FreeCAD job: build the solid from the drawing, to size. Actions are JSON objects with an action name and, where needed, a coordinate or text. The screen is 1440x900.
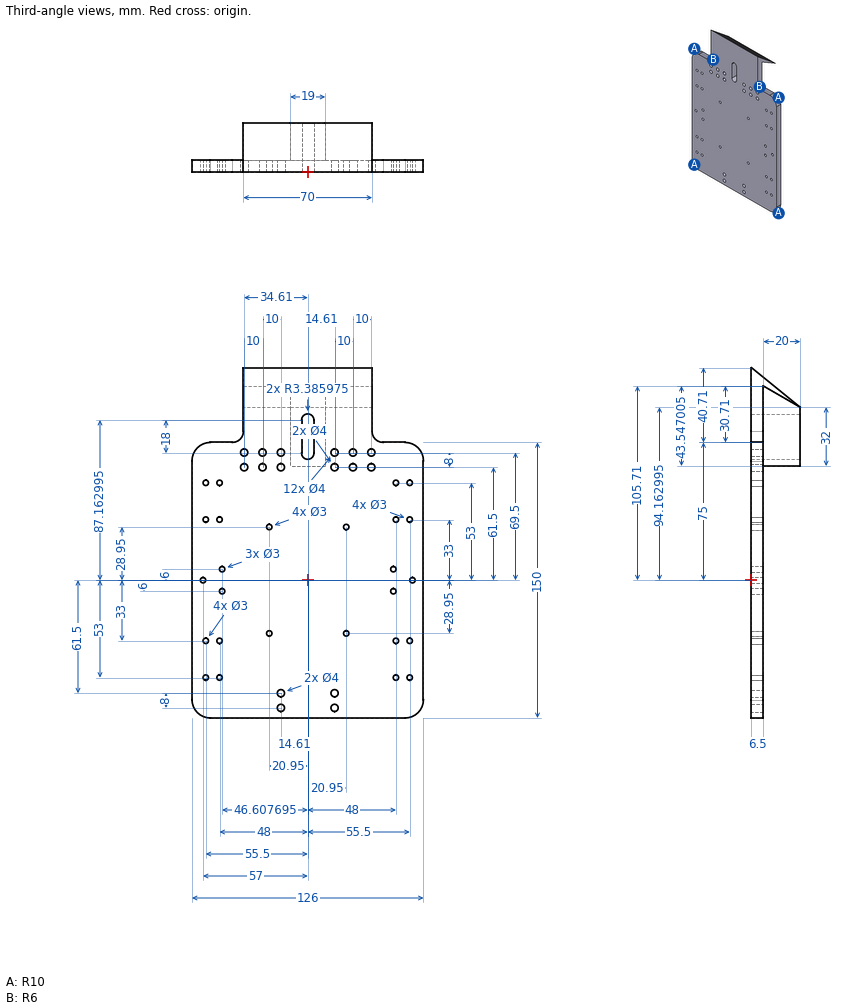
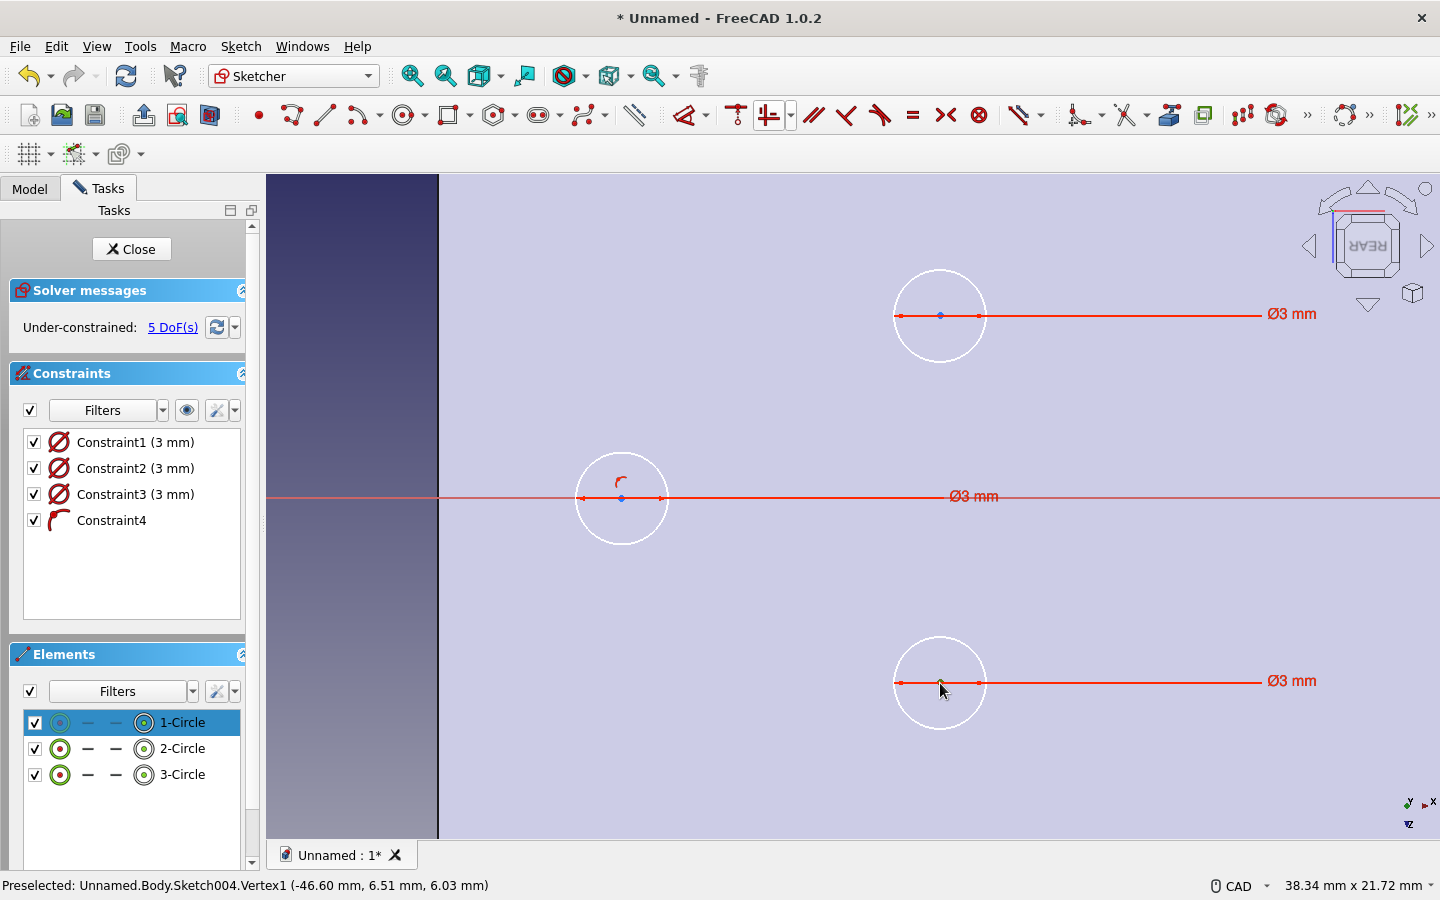
{"action": "left_click", "coordinate": [940, 316]}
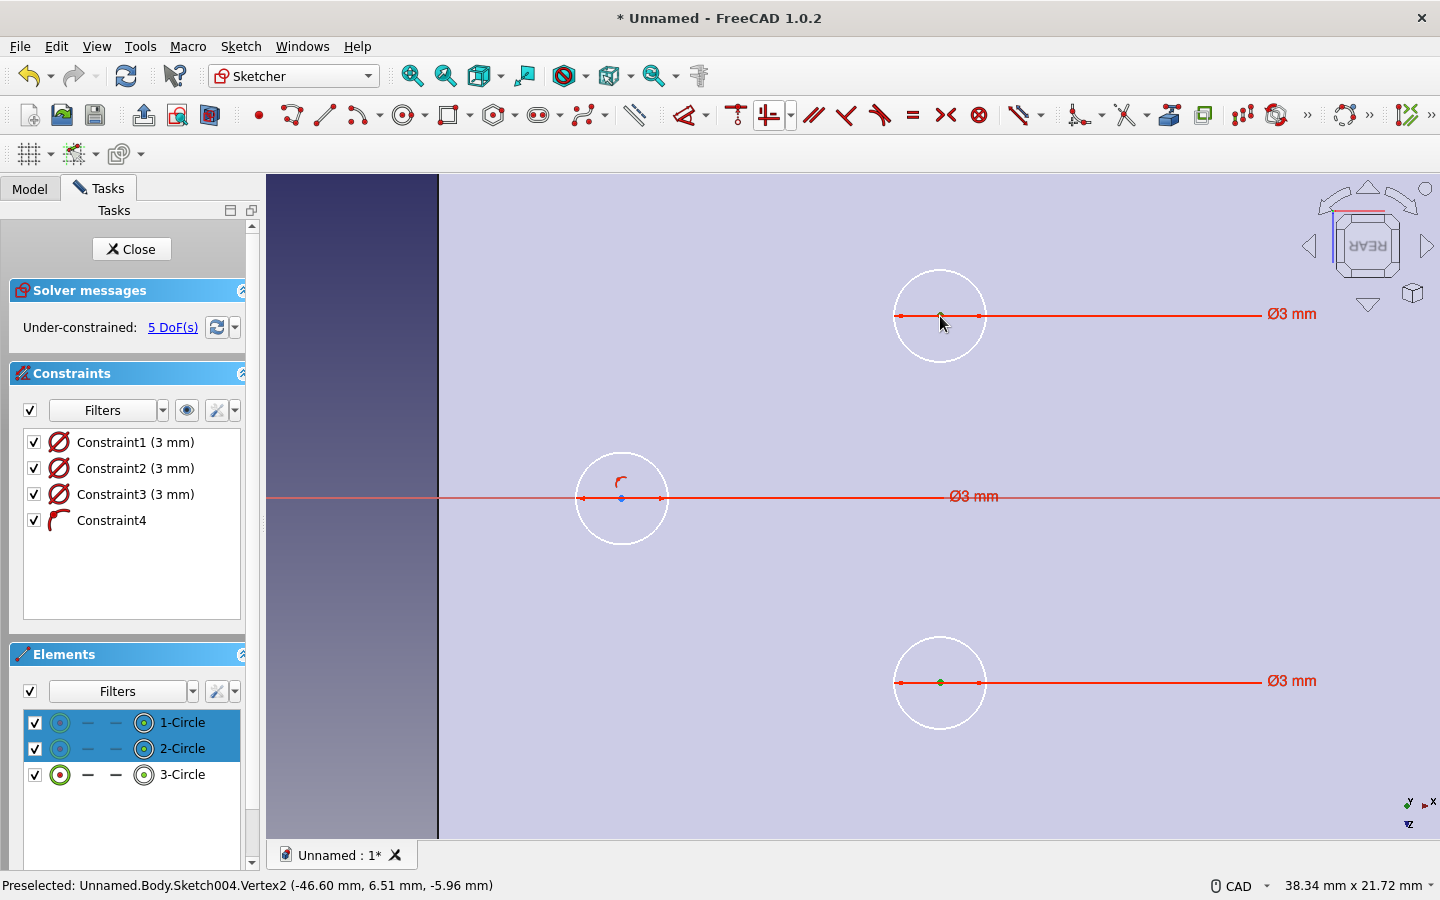
{"action": "key", "text": "v"}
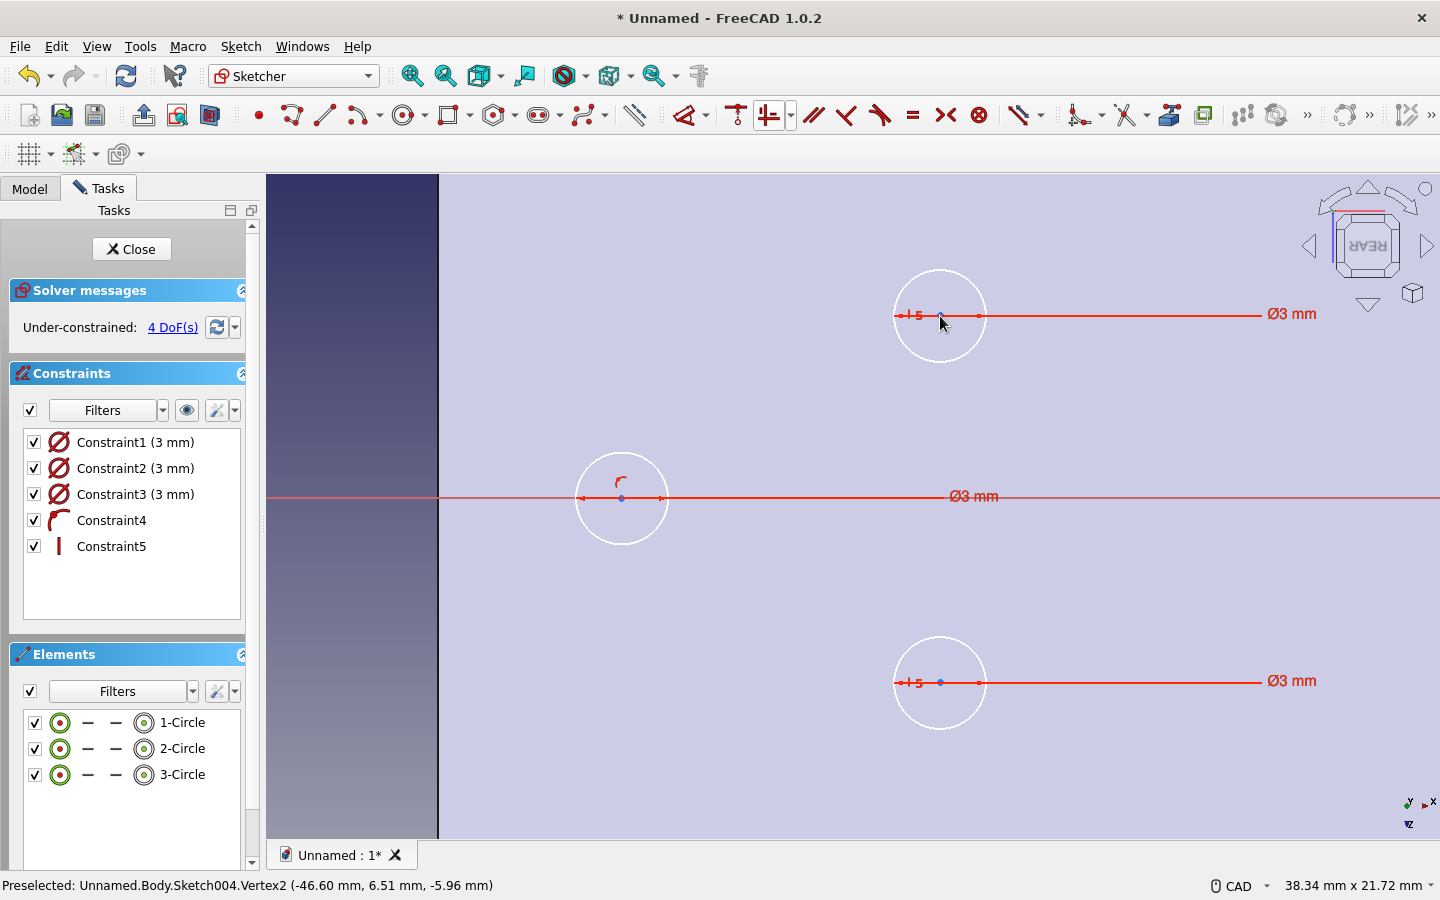
{"action": "left_click", "coordinate": [684, 116]}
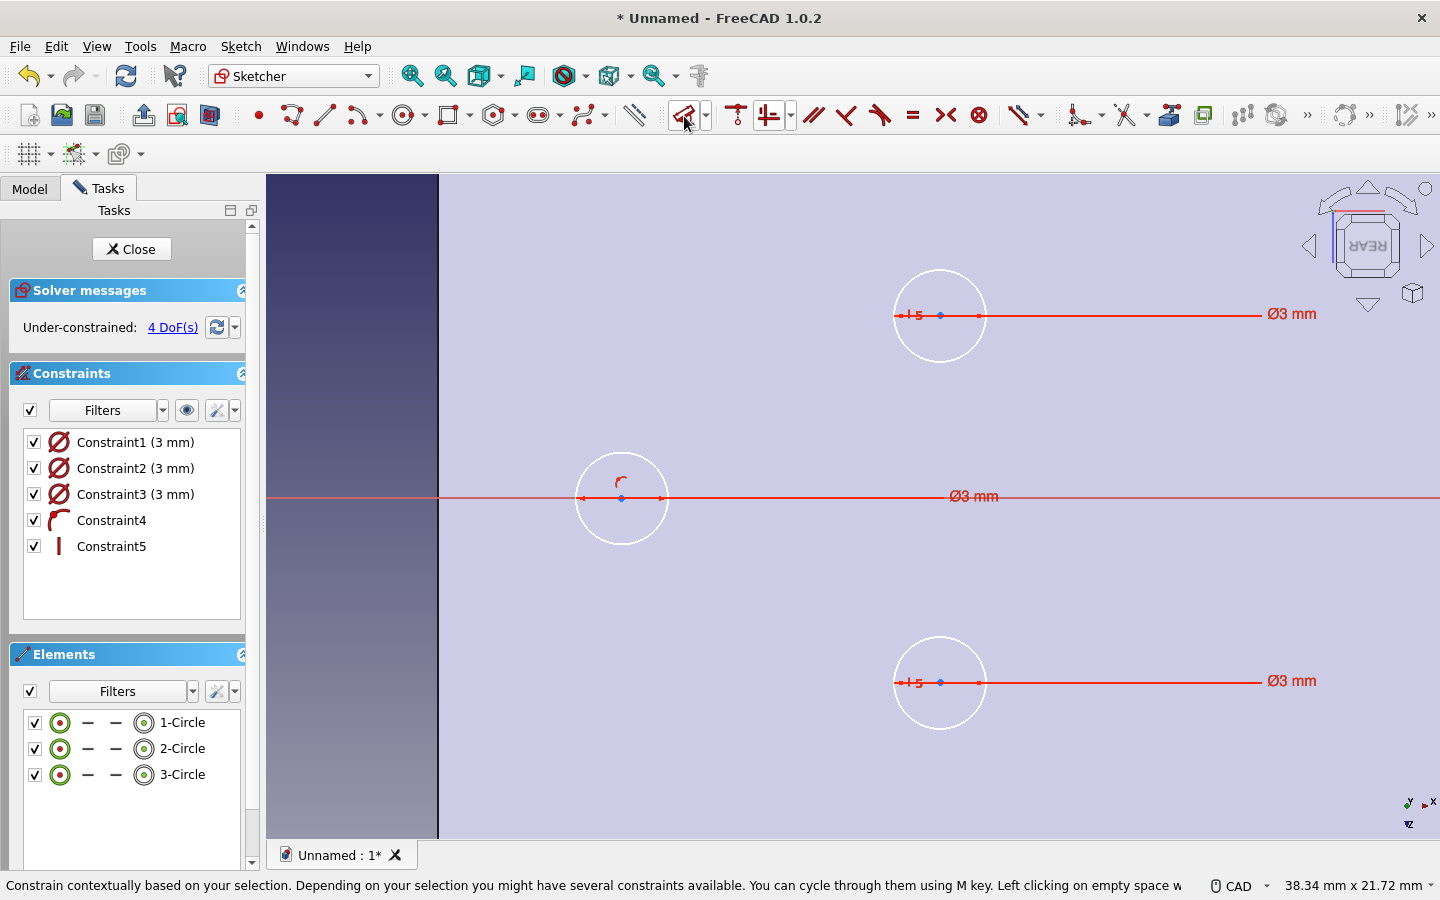
{"action": "left_click", "coordinate": [940, 683]}
{"action": "left_click", "coordinate": [906, 591]}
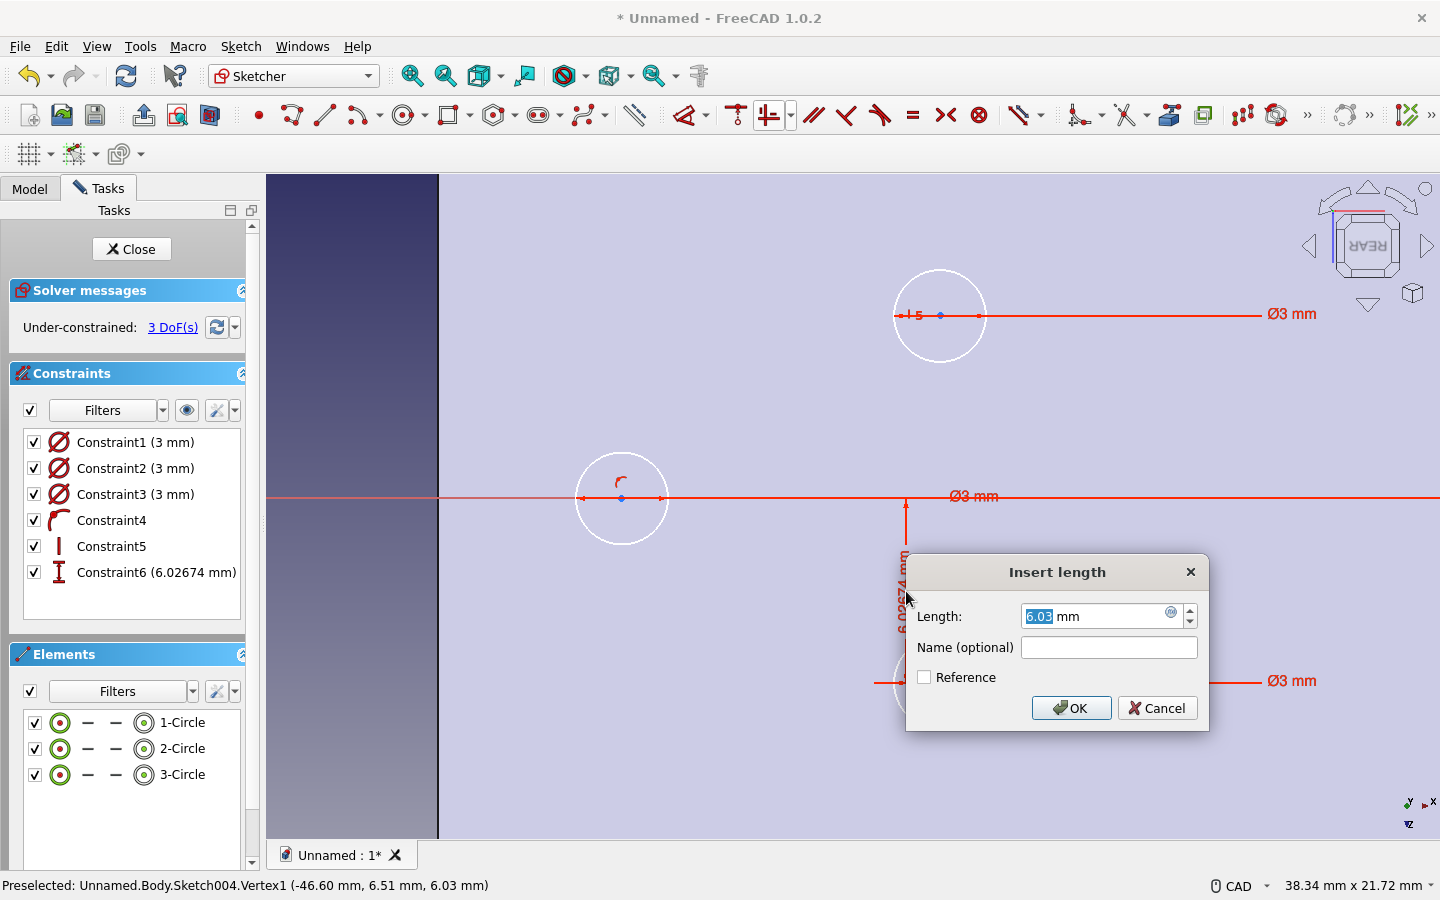
{"action": "type", "text": "6"}
{"action": "key", "text": "Return"}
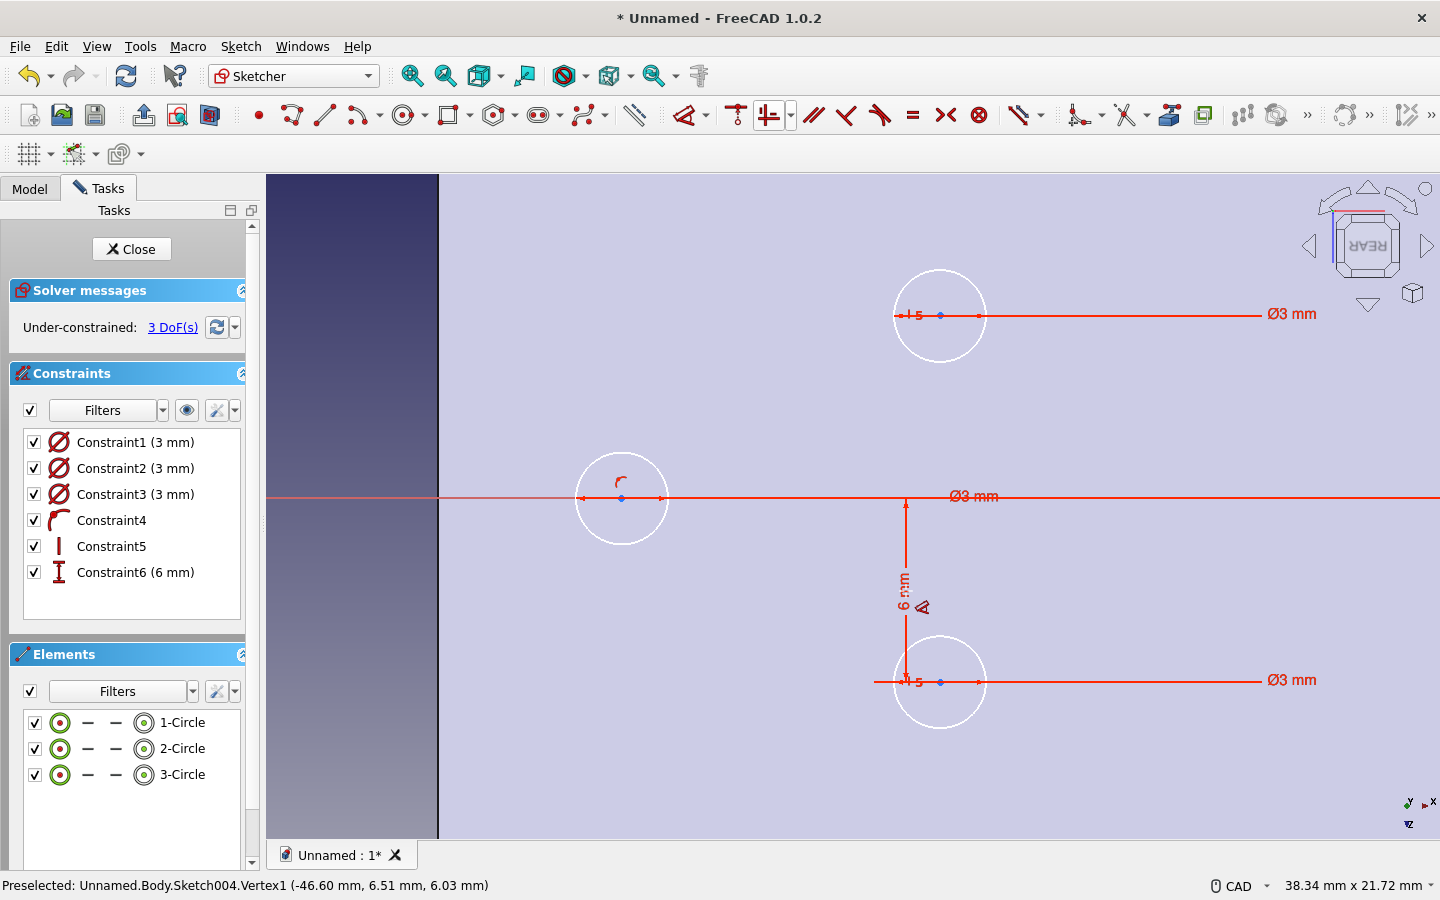
{"action": "left_click", "coordinate": [940, 316]}
{"action": "left_click", "coordinate": [906, 407]}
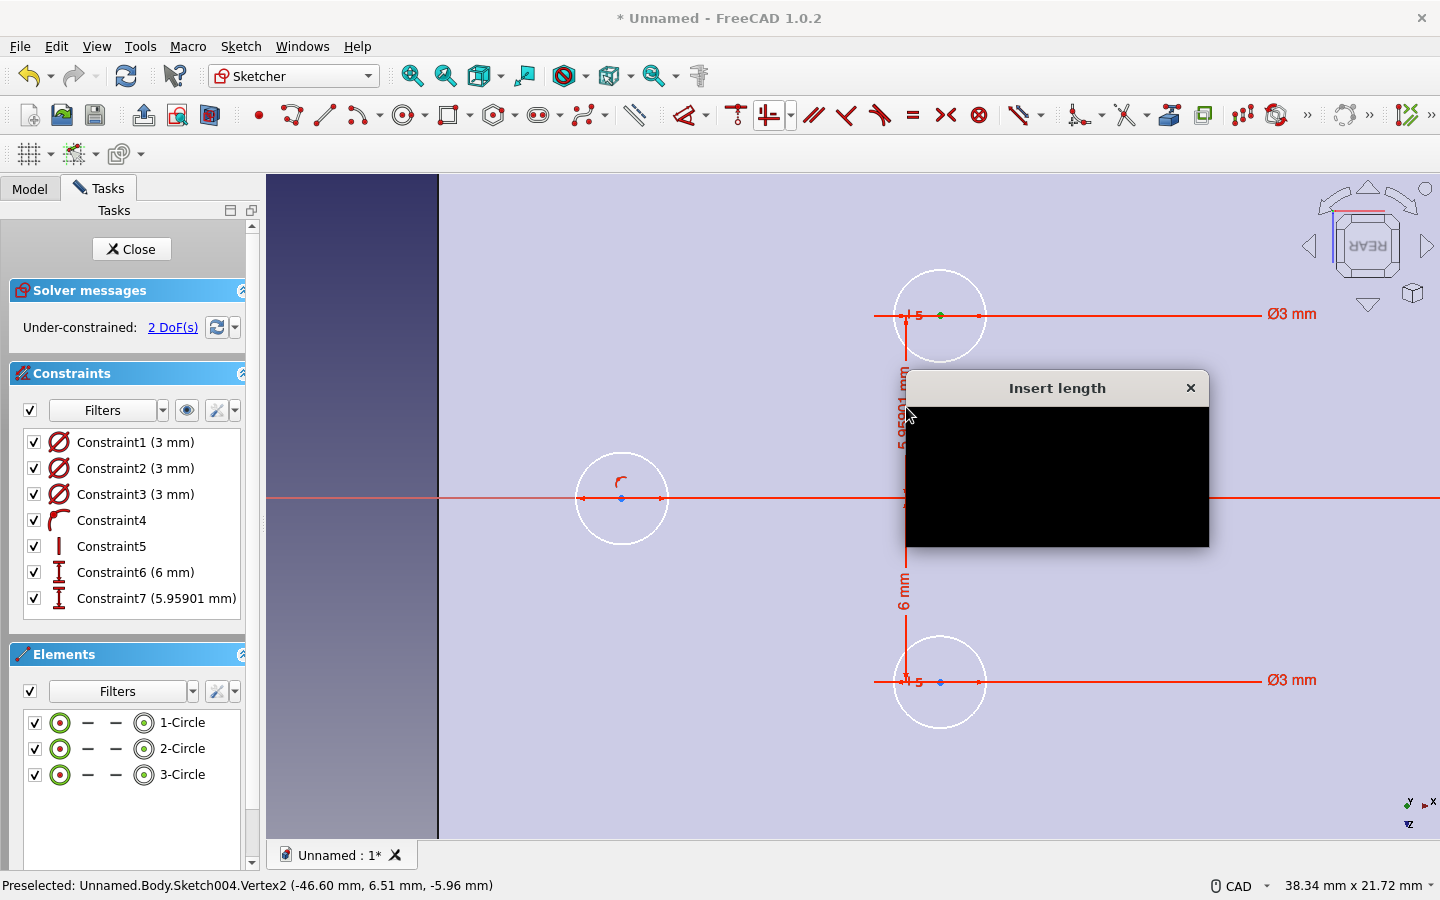
{"action": "type", "text": "6"}
{"action": "key", "text": "Return"}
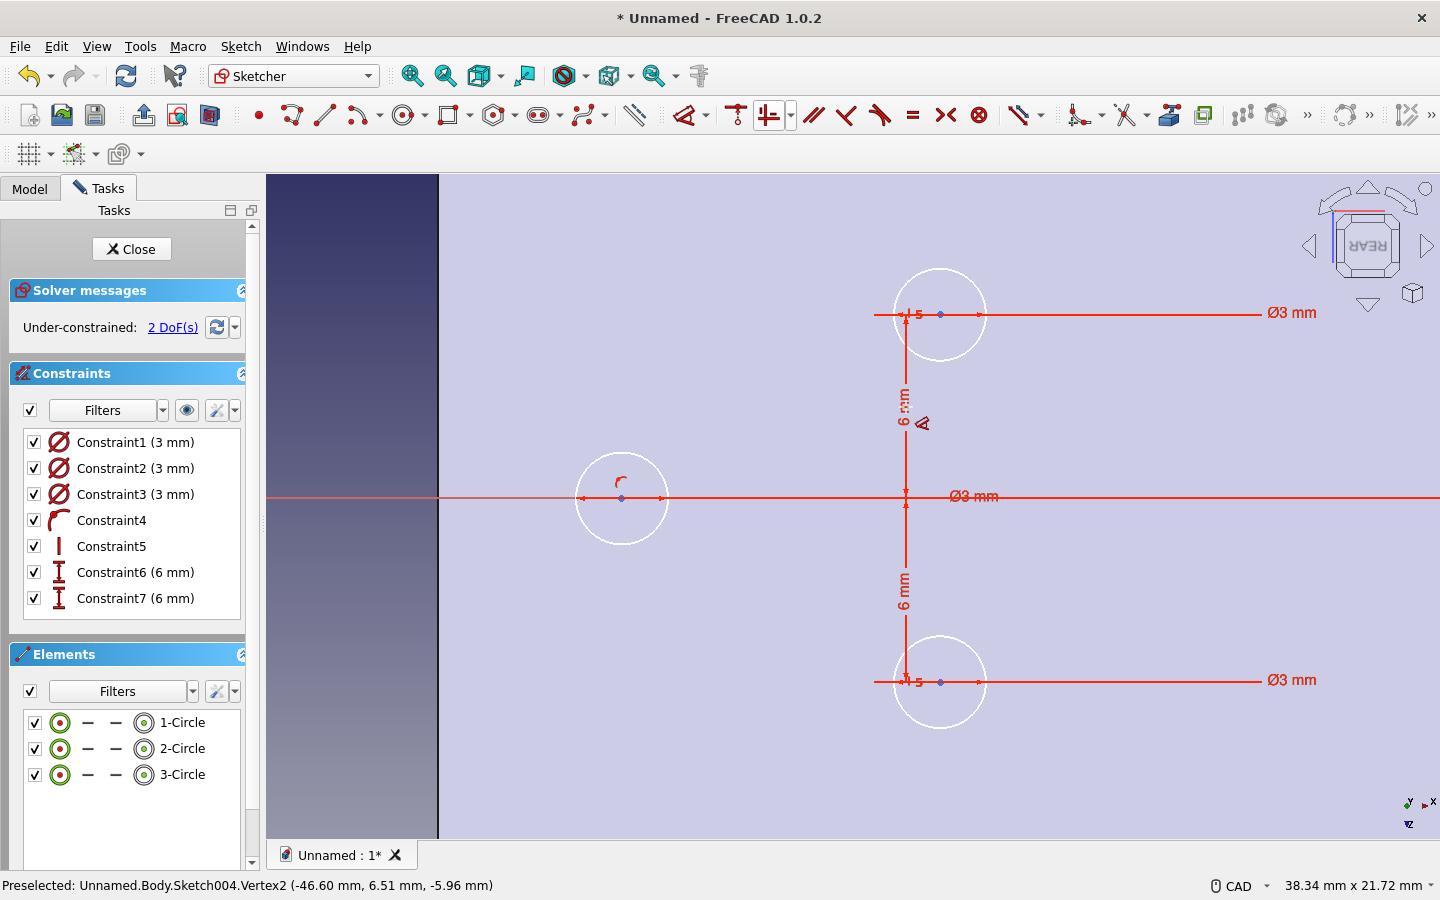
{"action": "left_click", "coordinate": [622, 498]}
{"action": "left_click", "coordinate": [948, 532]}